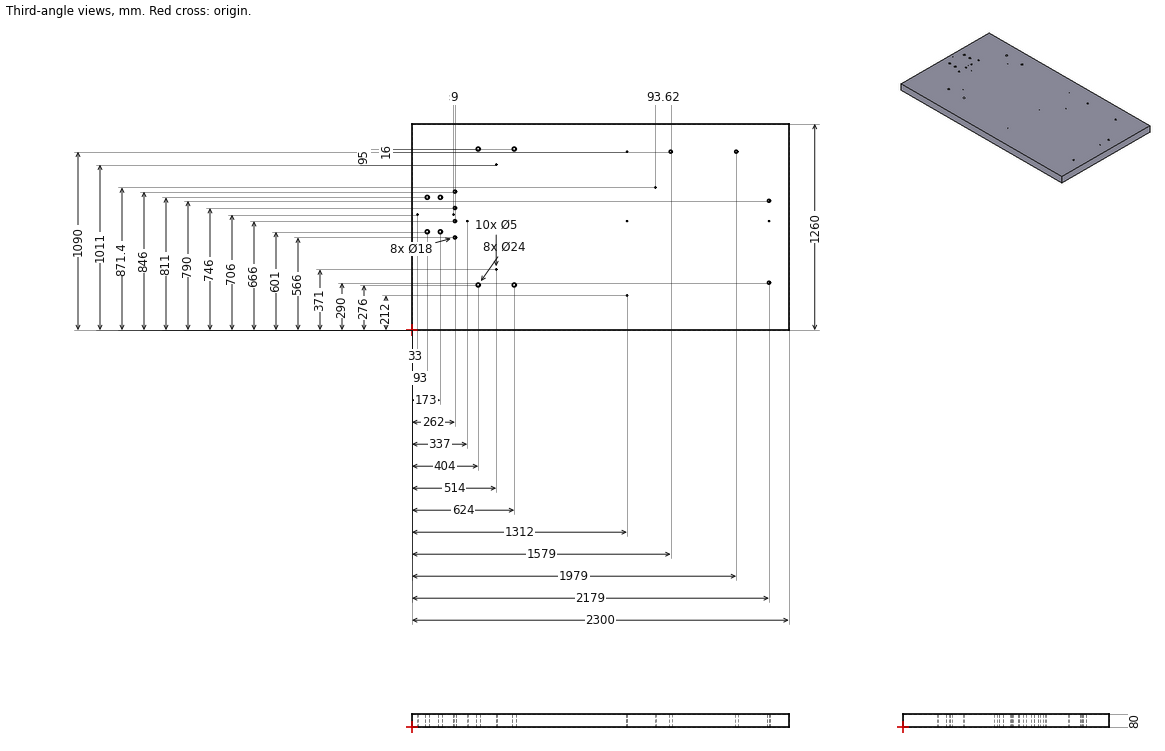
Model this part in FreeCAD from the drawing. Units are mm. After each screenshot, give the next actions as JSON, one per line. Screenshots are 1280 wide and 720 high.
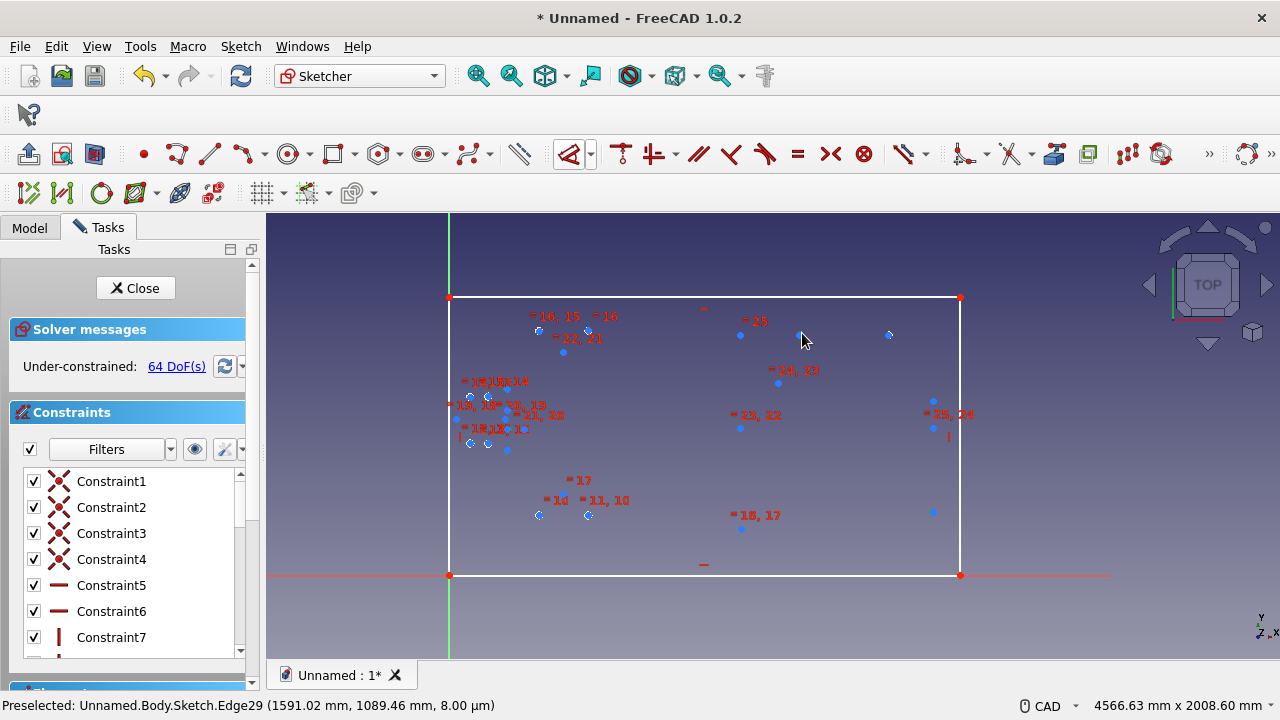
{"action": "scroll", "coordinate": [891, 333], "scroll_direction": "up", "scroll_amount": 8}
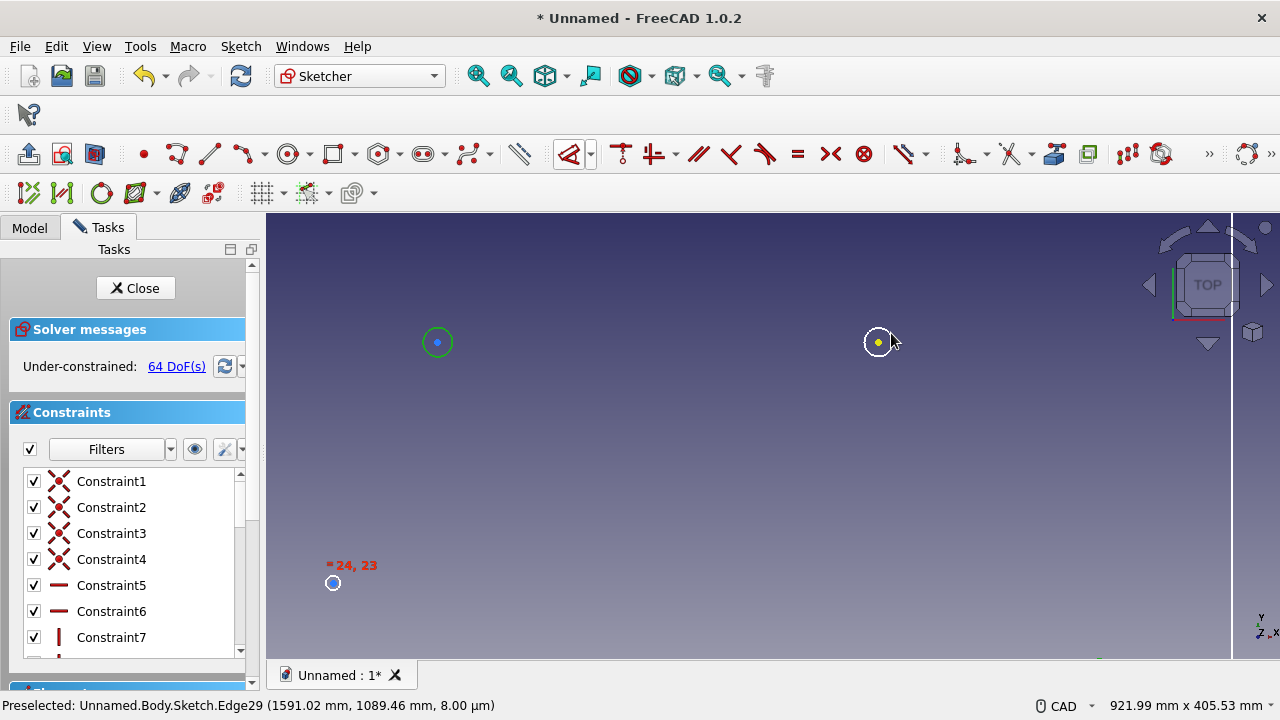
{"action": "left_click", "coordinate": [889, 332]}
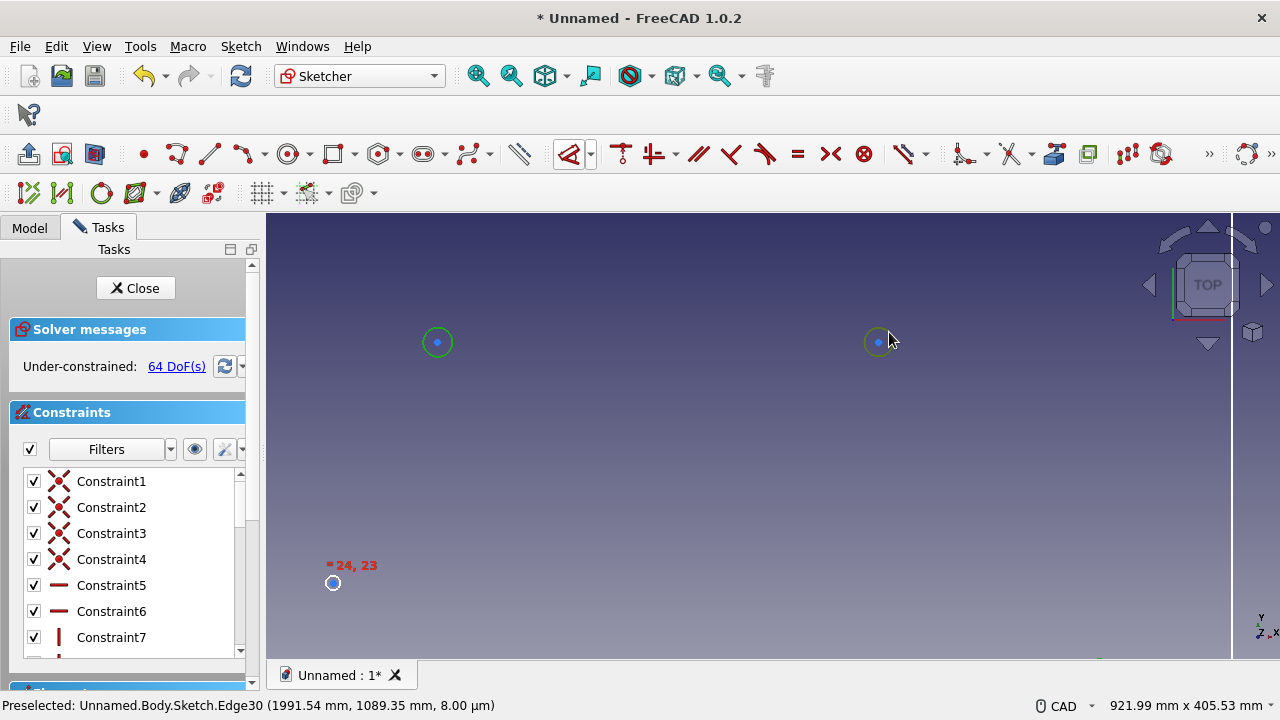
{"action": "left_click", "coordinate": [798, 154]}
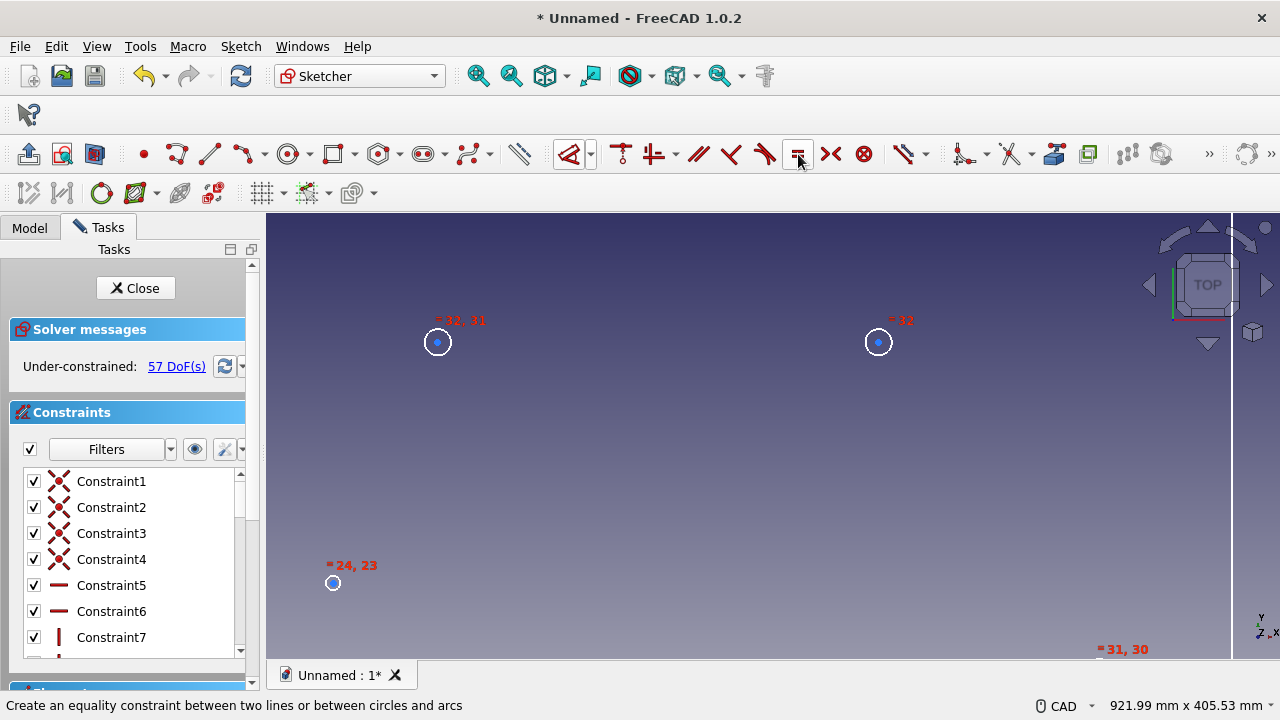
{"action": "left_click", "coordinate": [568, 154]}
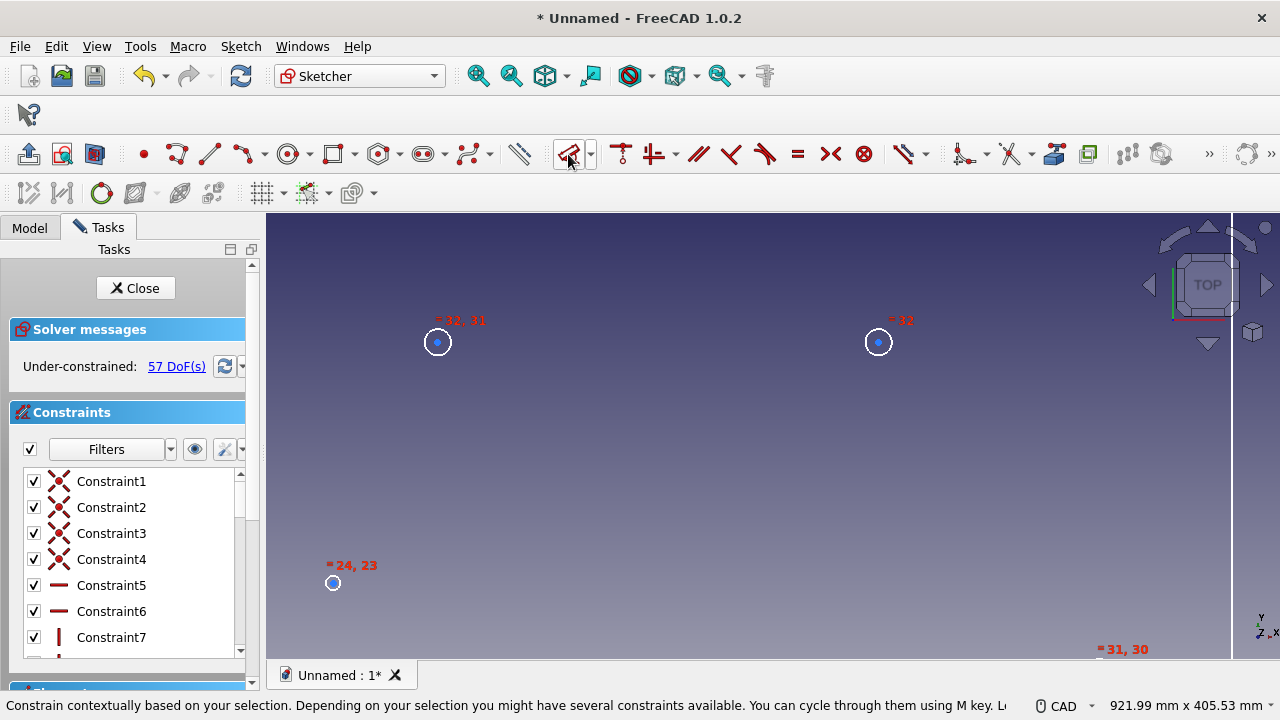
{"action": "scroll", "coordinate": [891, 333], "scroll_direction": "down", "scroll_amount": 8}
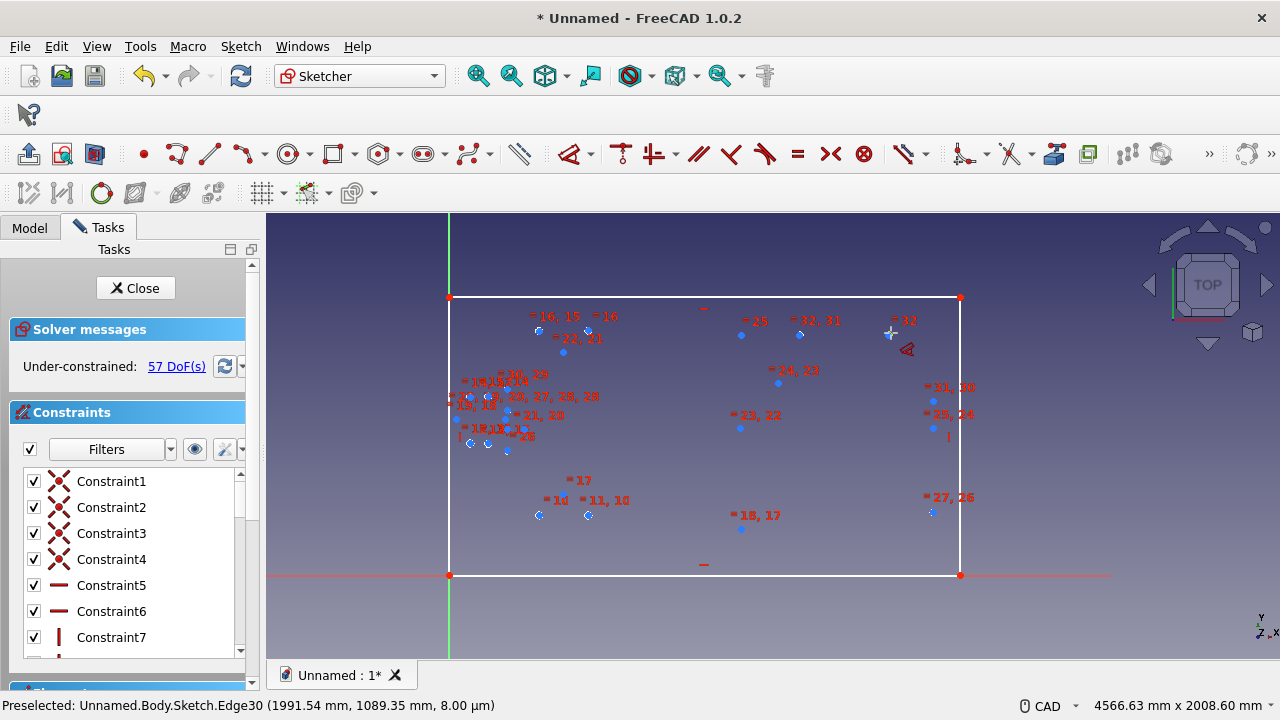
{"action": "scroll", "coordinate": [542, 513], "scroll_direction": "up", "scroll_amount": 11}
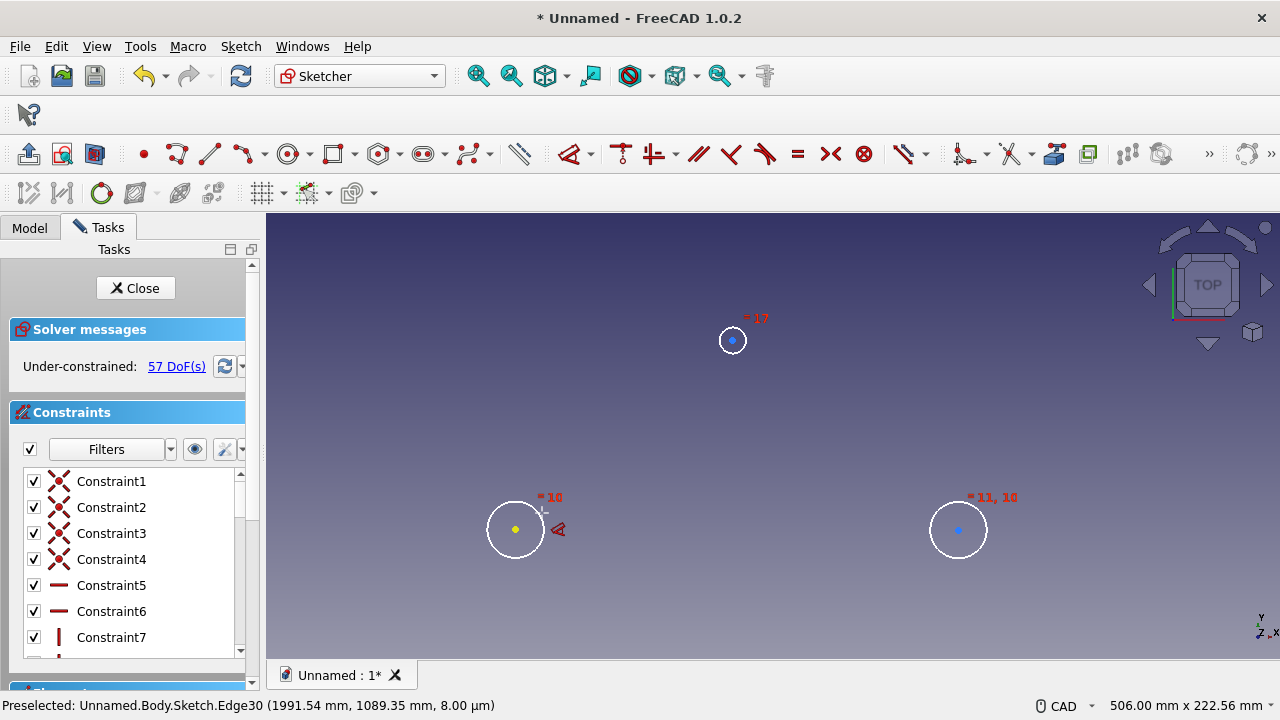
{"action": "left_click", "coordinate": [535, 510]}
{"action": "left_click", "coordinate": [557, 487]}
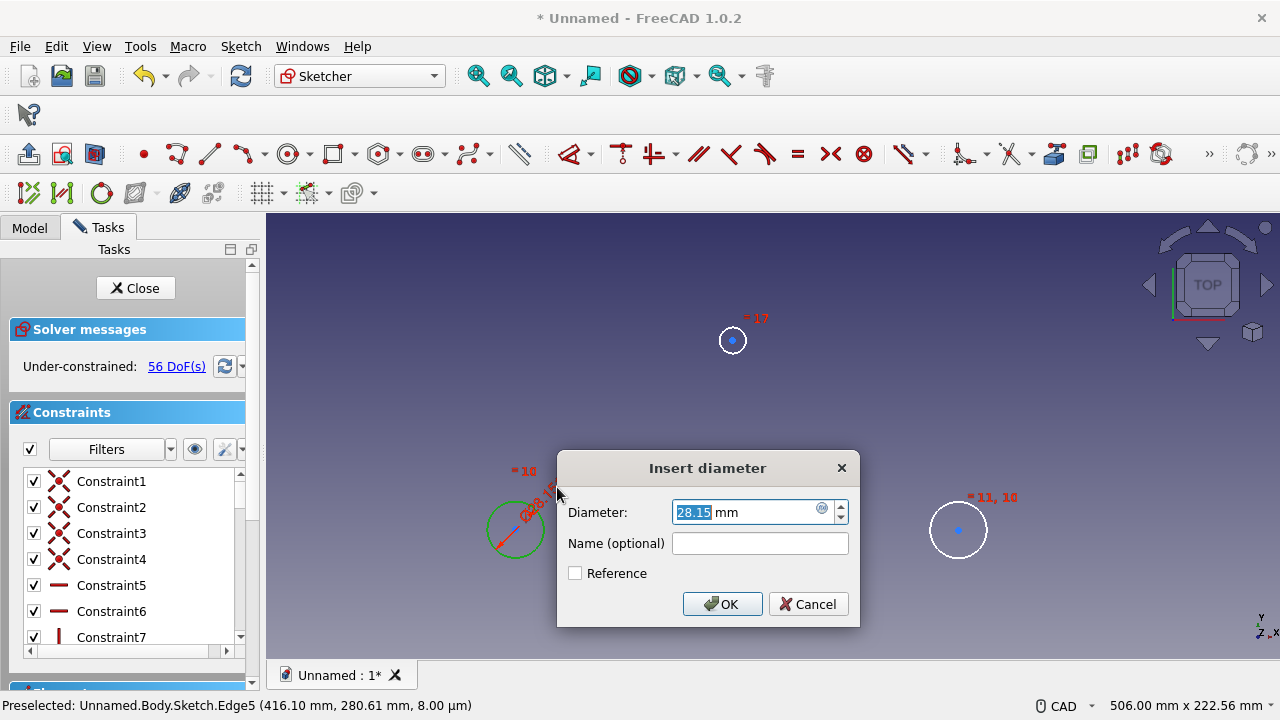
{"action": "type", "text": "24"}
{"action": "key", "text": "Return"}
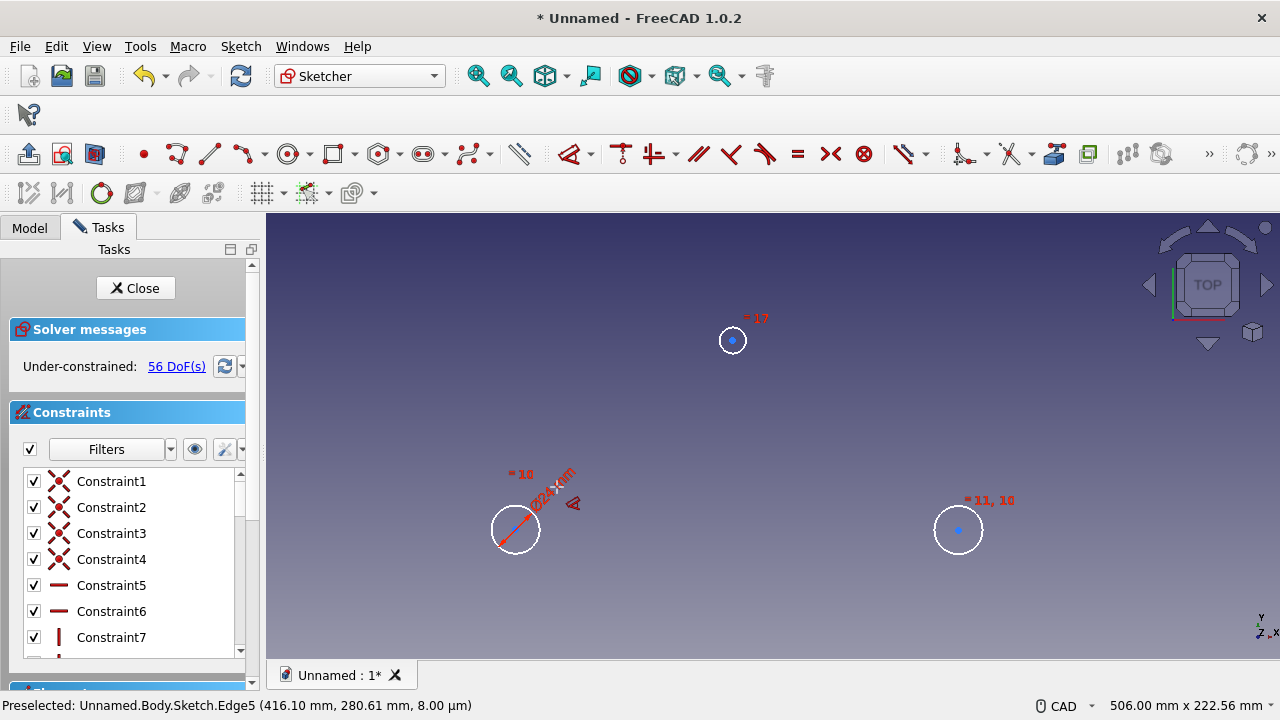
{"action": "scroll", "coordinate": [742, 331], "scroll_direction": "up", "scroll_amount": 7}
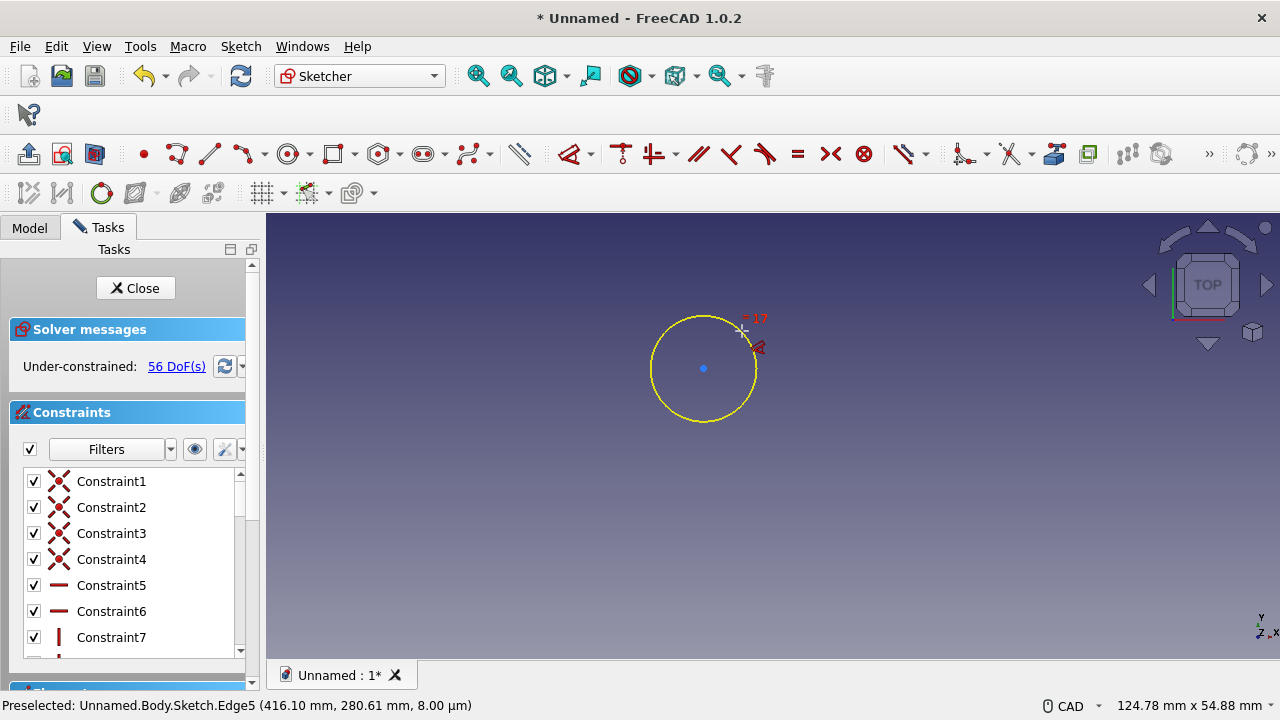
{"action": "left_click", "coordinate": [741, 331]}
{"action": "left_click", "coordinate": [764, 308]}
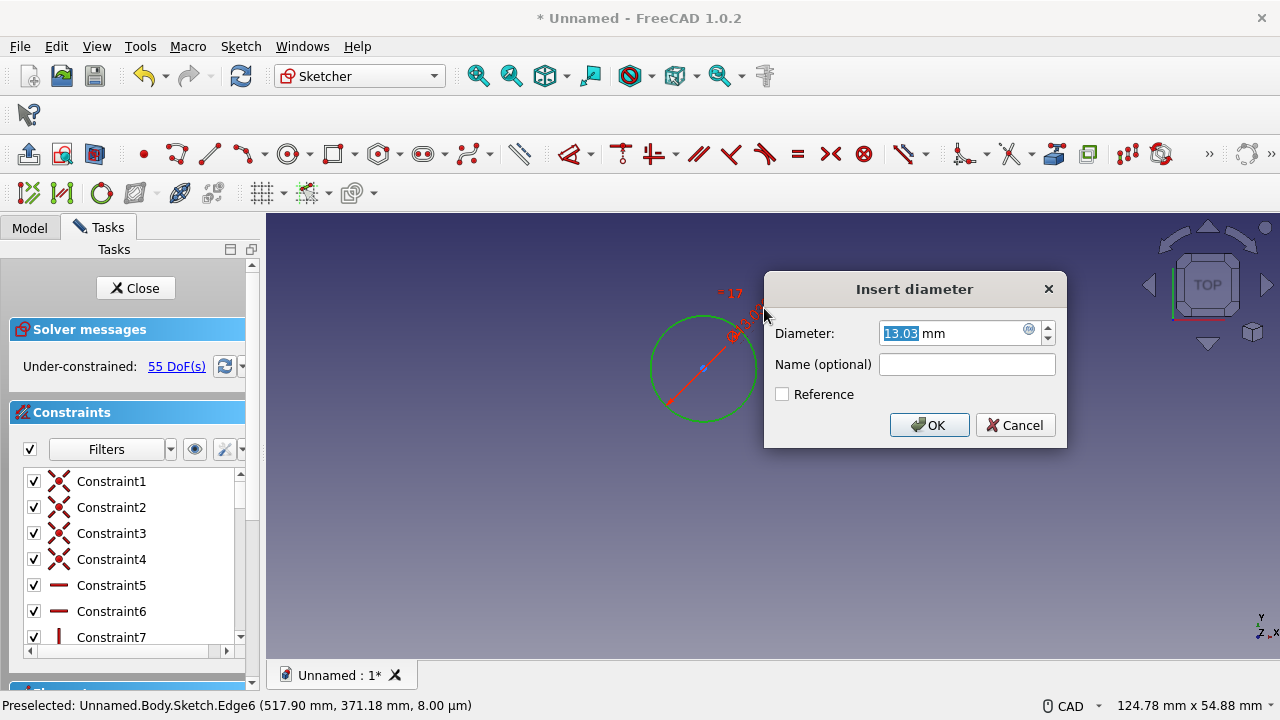
{"action": "type", "text": "5"}
{"action": "key", "text": "Return"}